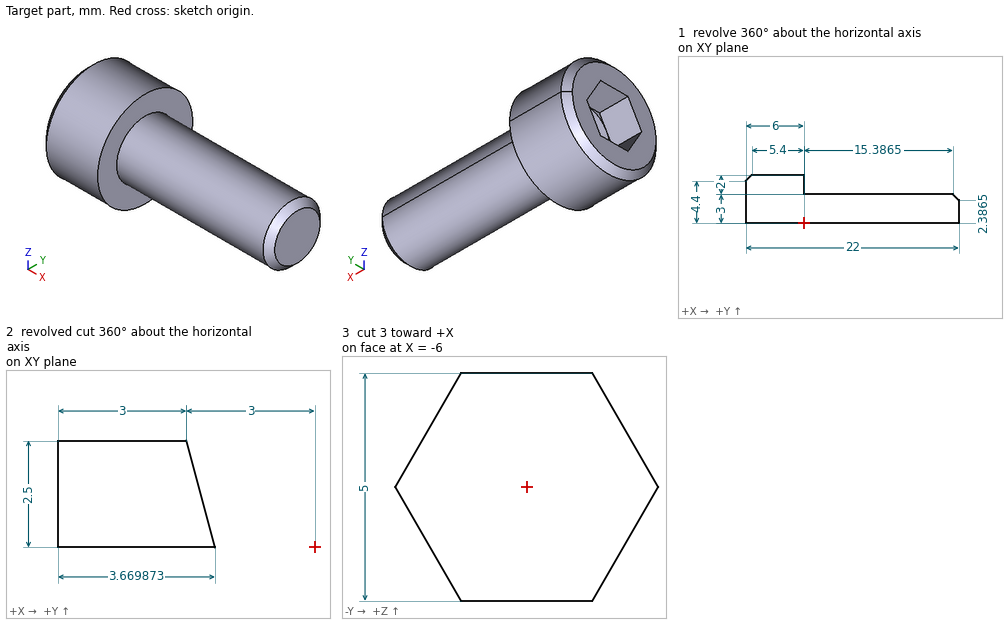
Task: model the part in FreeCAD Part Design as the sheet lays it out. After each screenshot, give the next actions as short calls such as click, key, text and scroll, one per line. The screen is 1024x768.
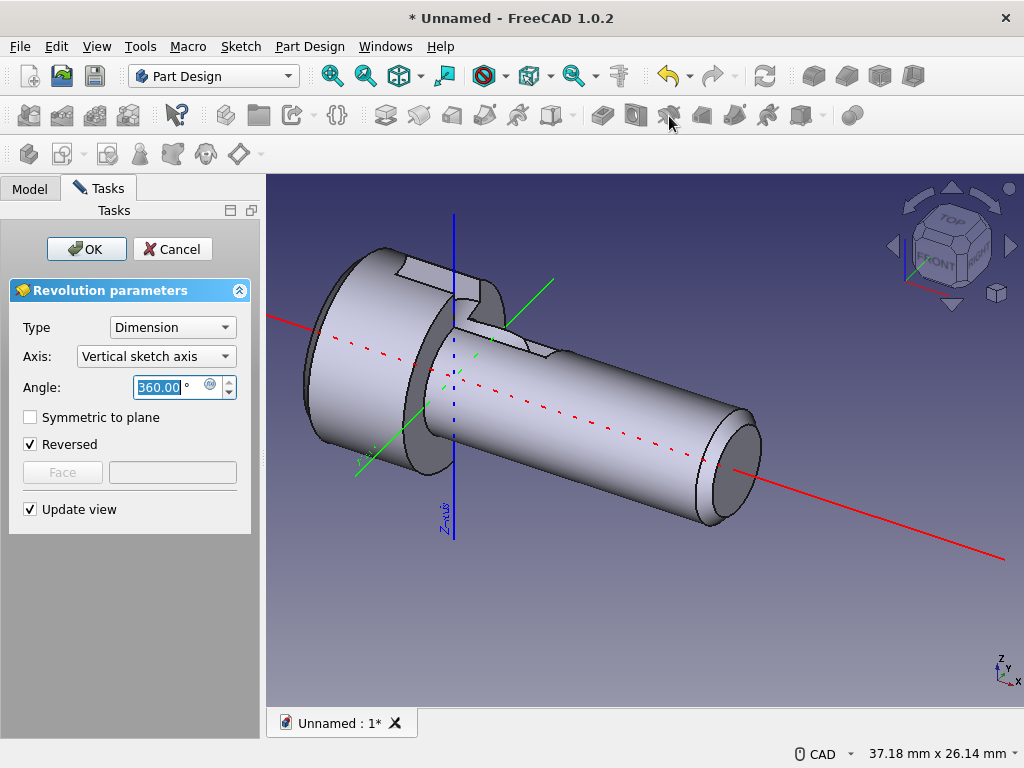
click(157, 356)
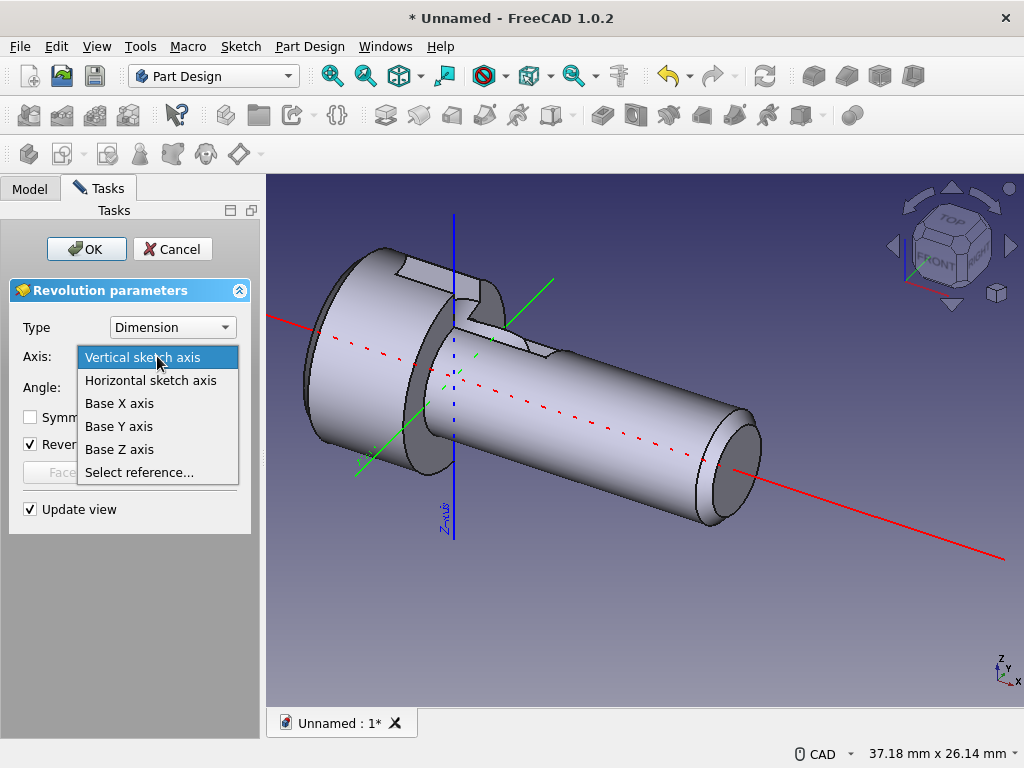
click(156, 380)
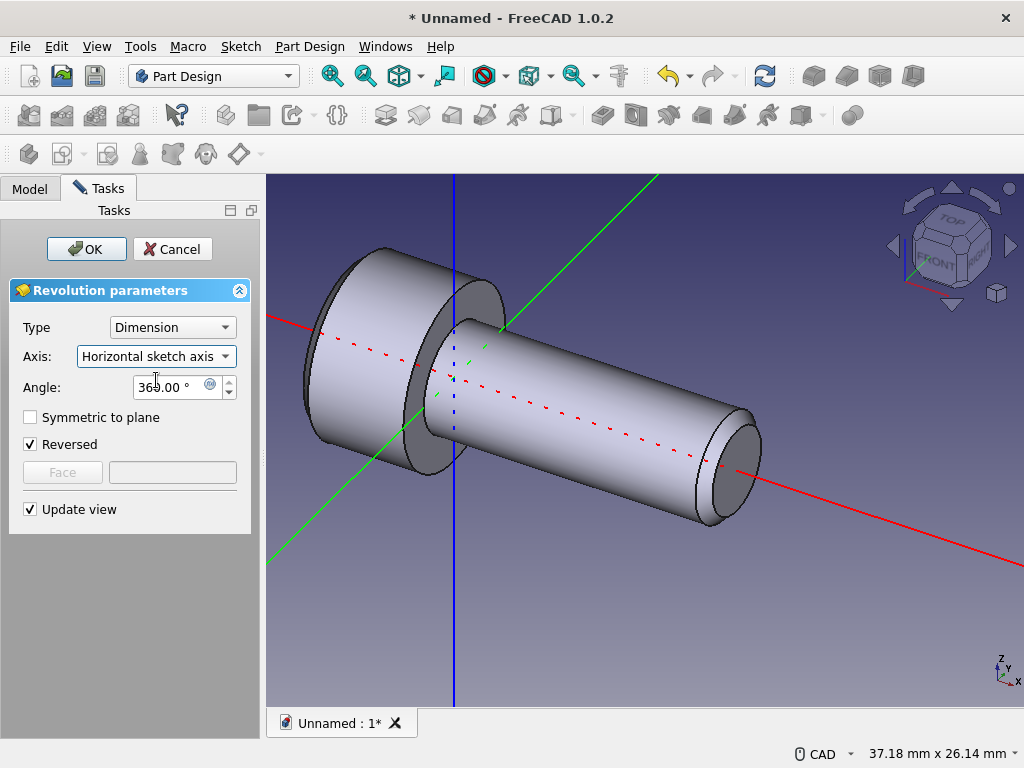
click(87, 249)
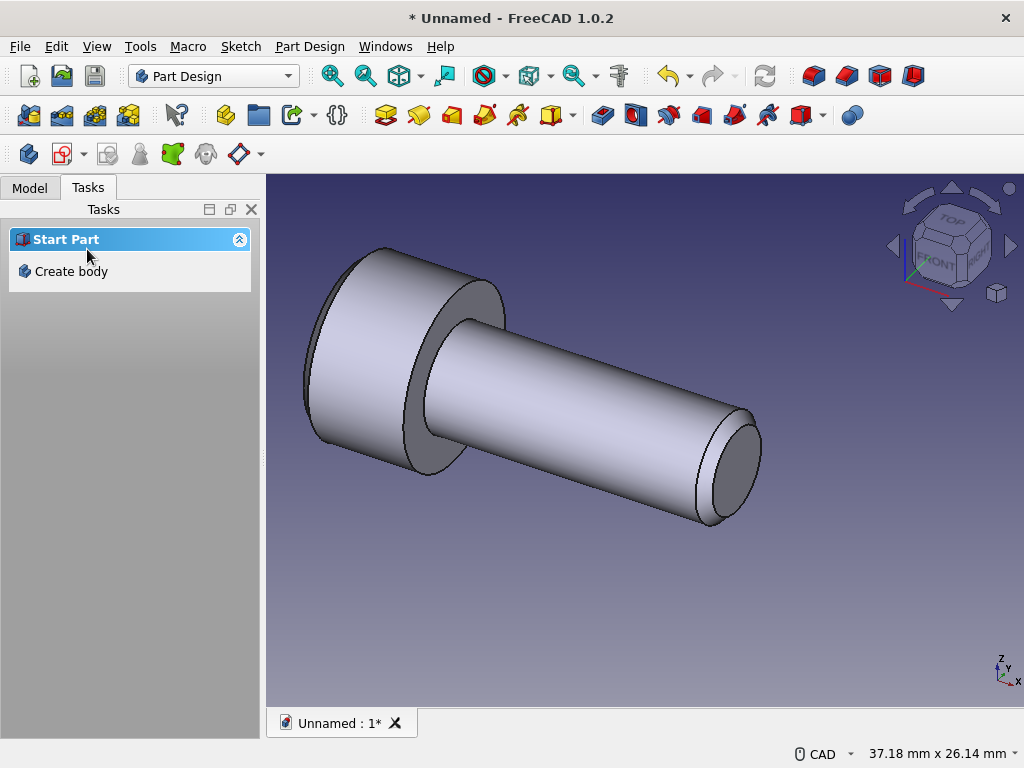
key(6)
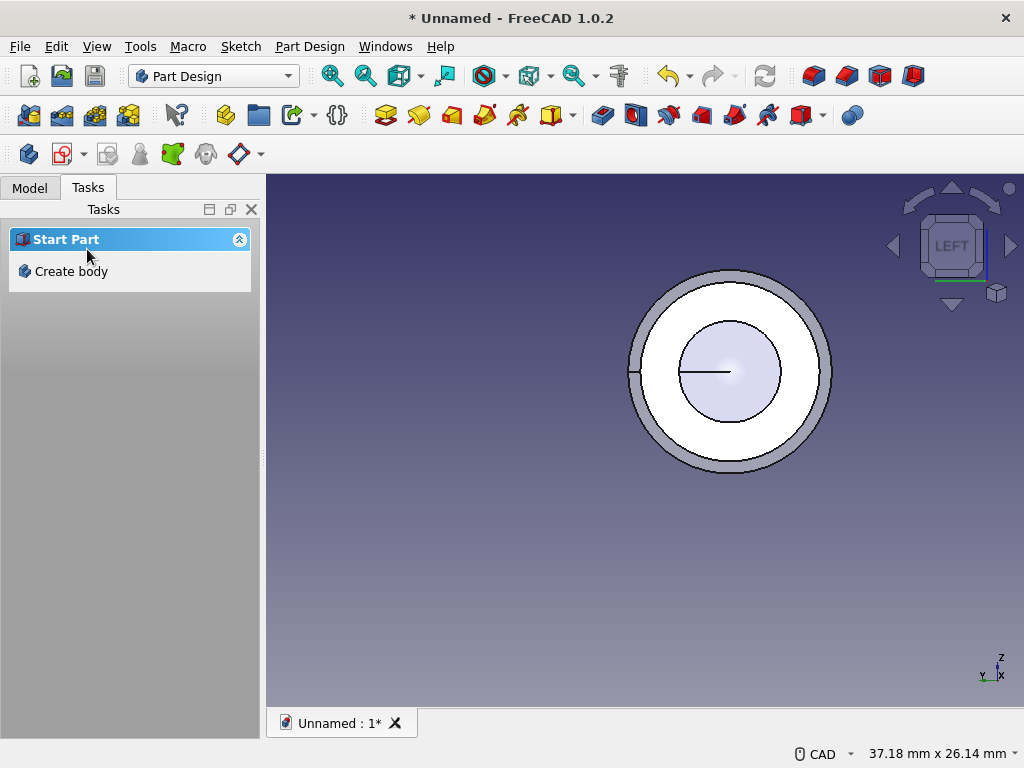
click(333, 76)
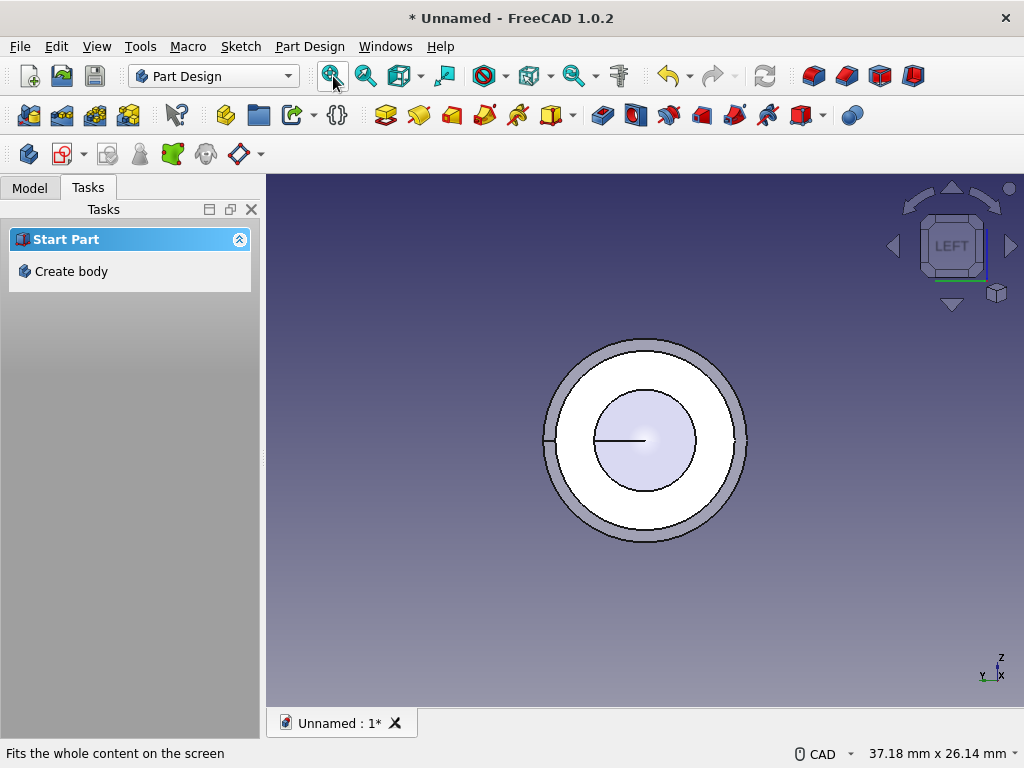
click(696, 491)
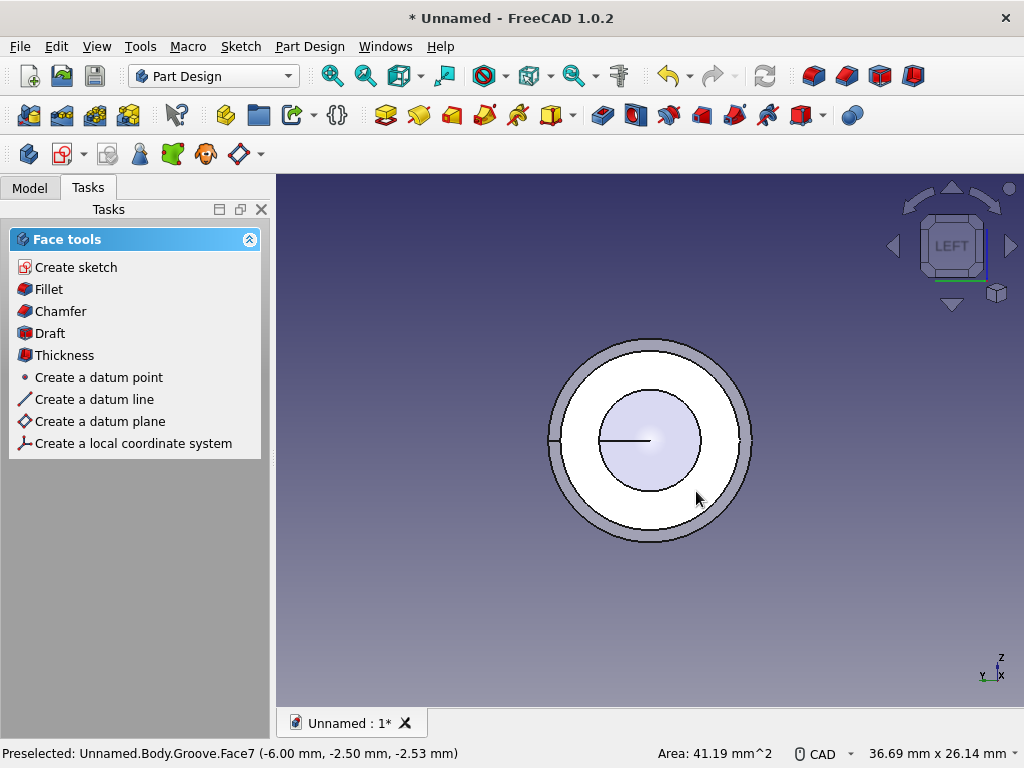
click(62, 154)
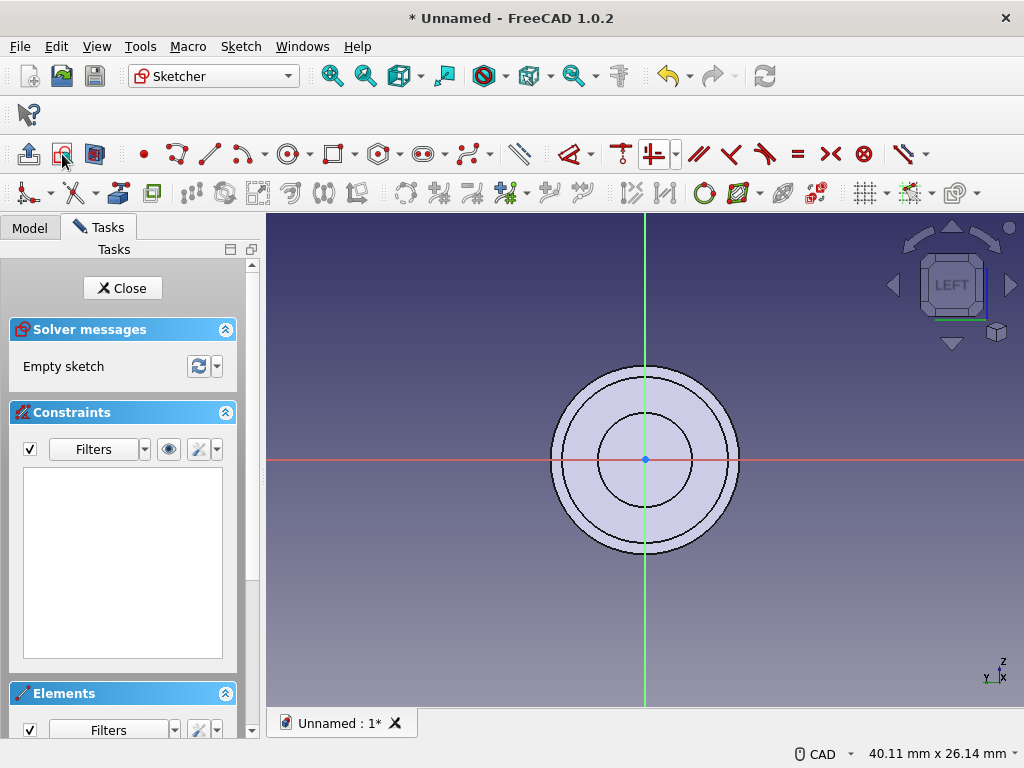
scroll(675, 460, up, 6)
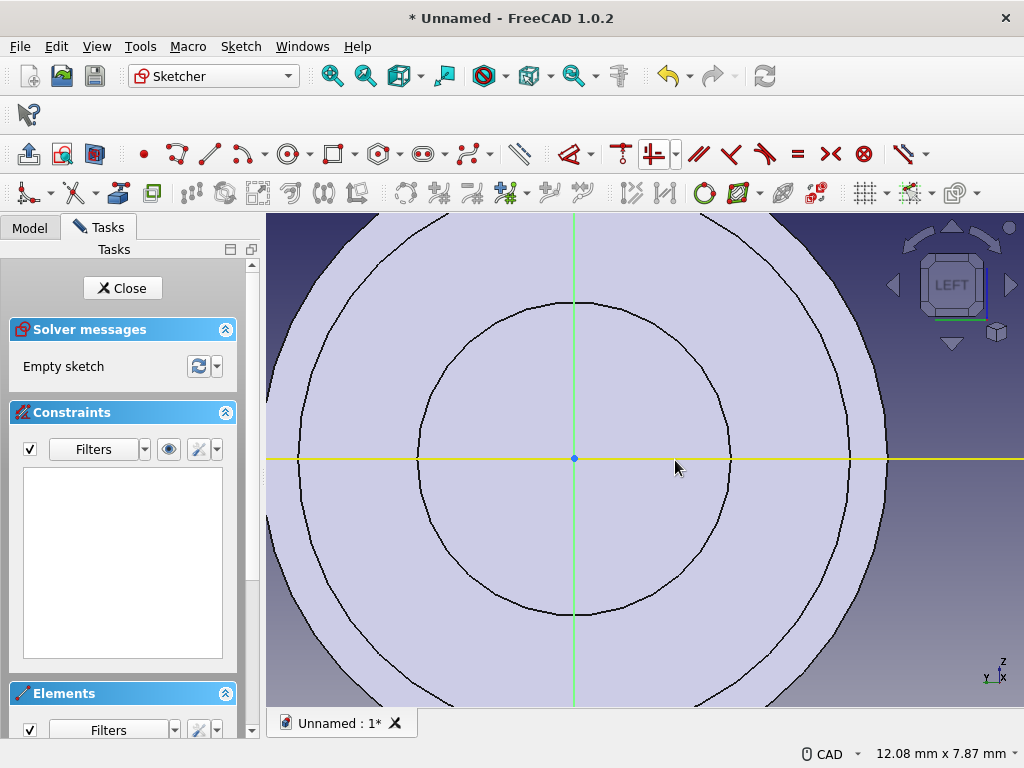
click(378, 154)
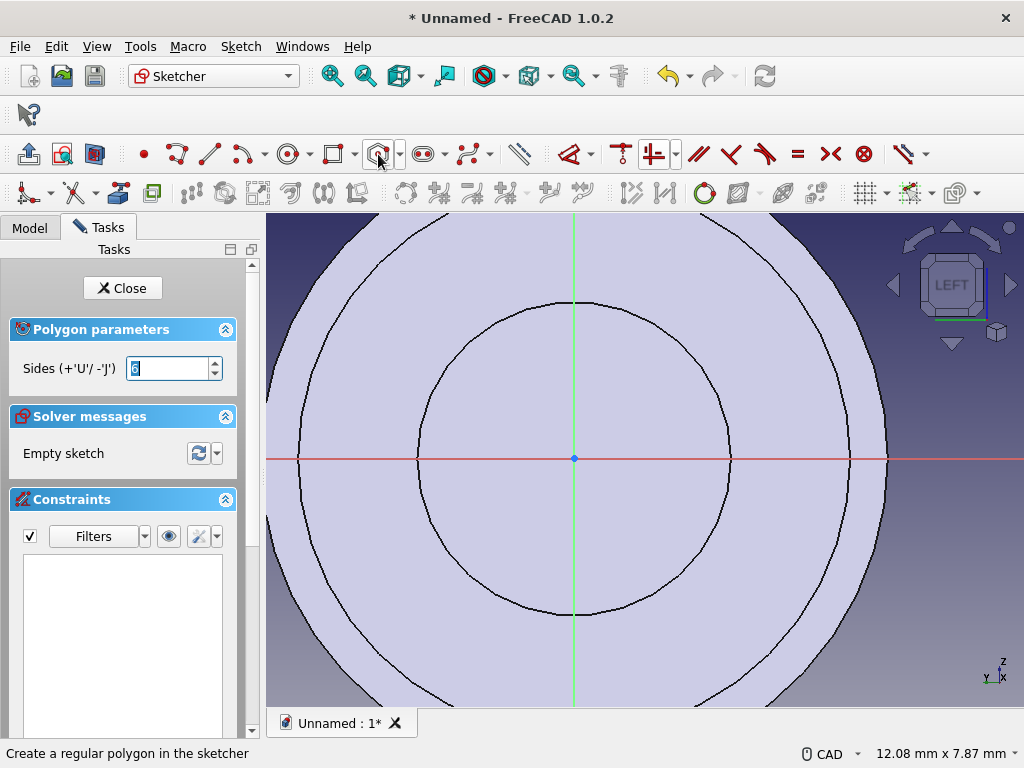
click(574, 459)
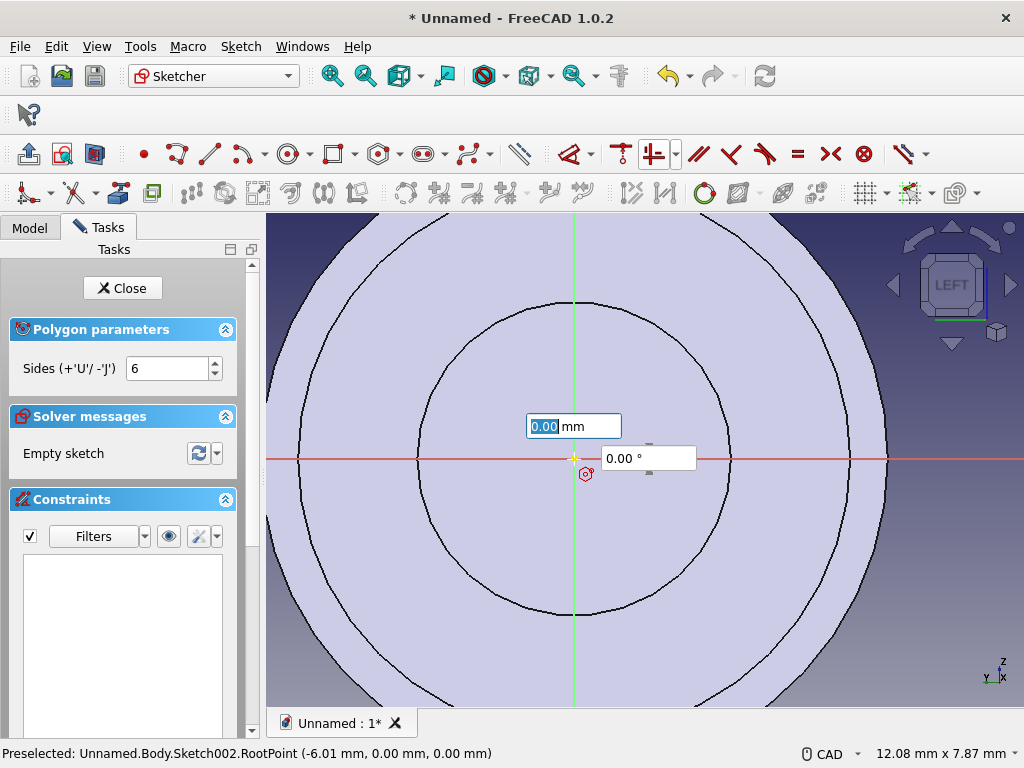
click(755, 459)
right_click(755, 459)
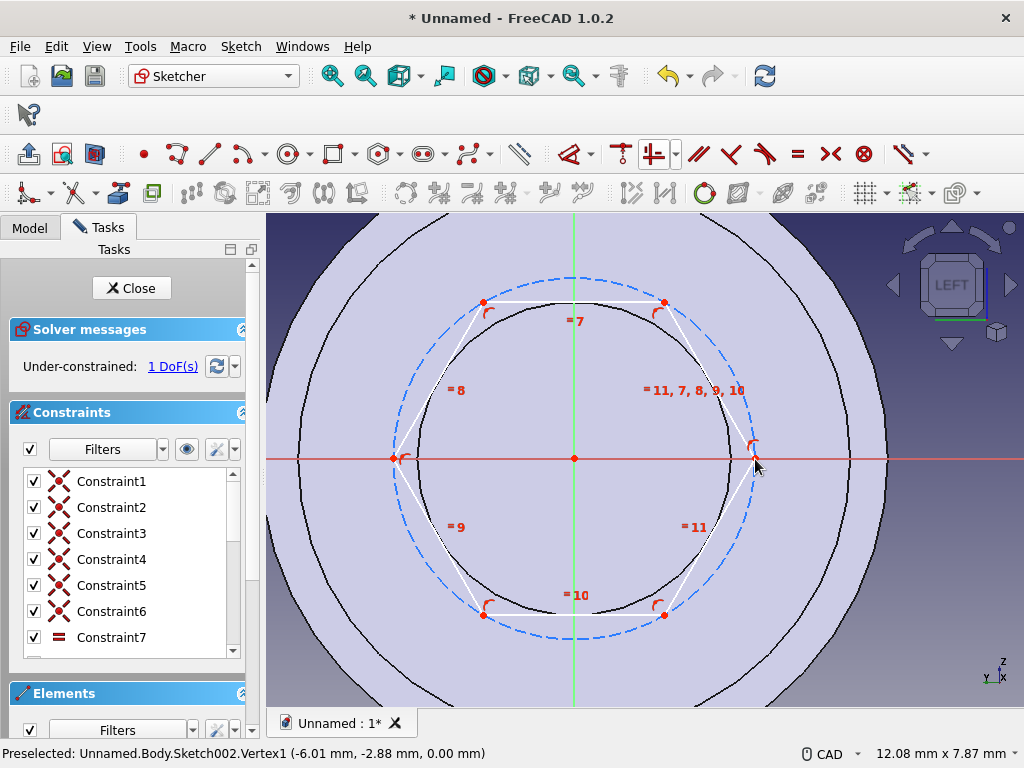
click(568, 154)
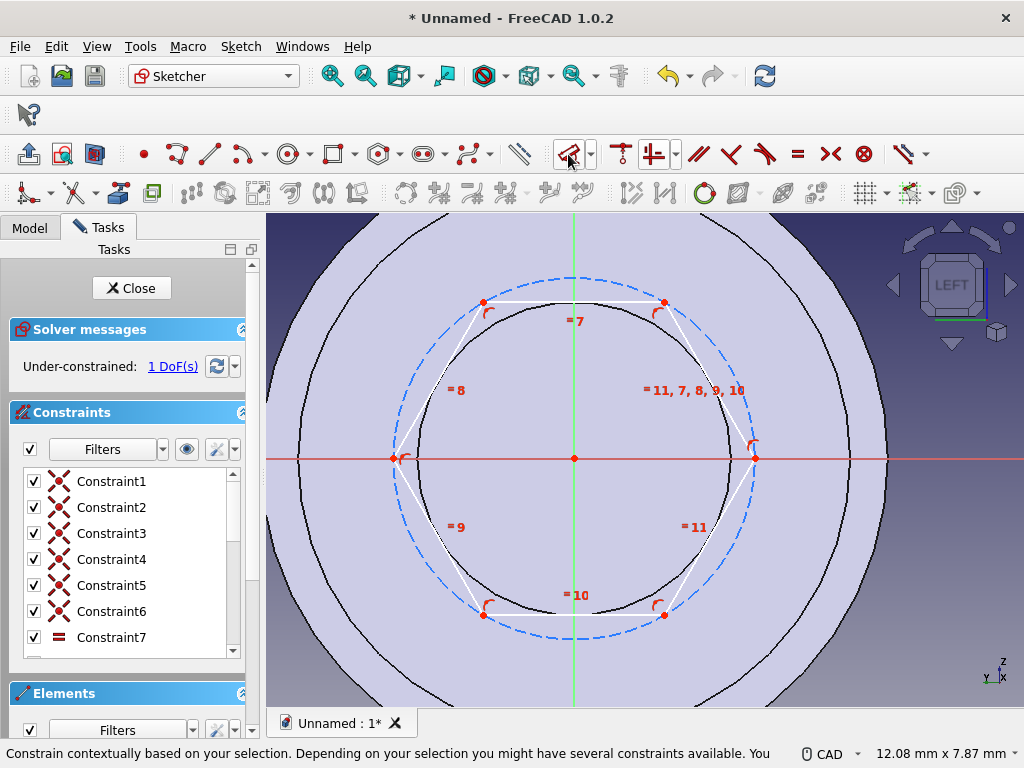
click(484, 615)